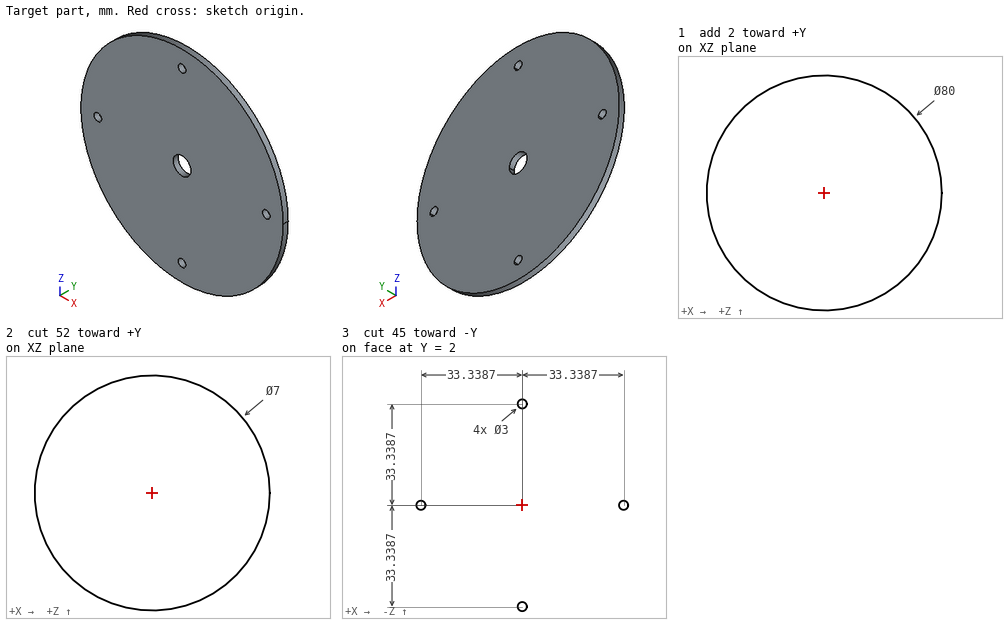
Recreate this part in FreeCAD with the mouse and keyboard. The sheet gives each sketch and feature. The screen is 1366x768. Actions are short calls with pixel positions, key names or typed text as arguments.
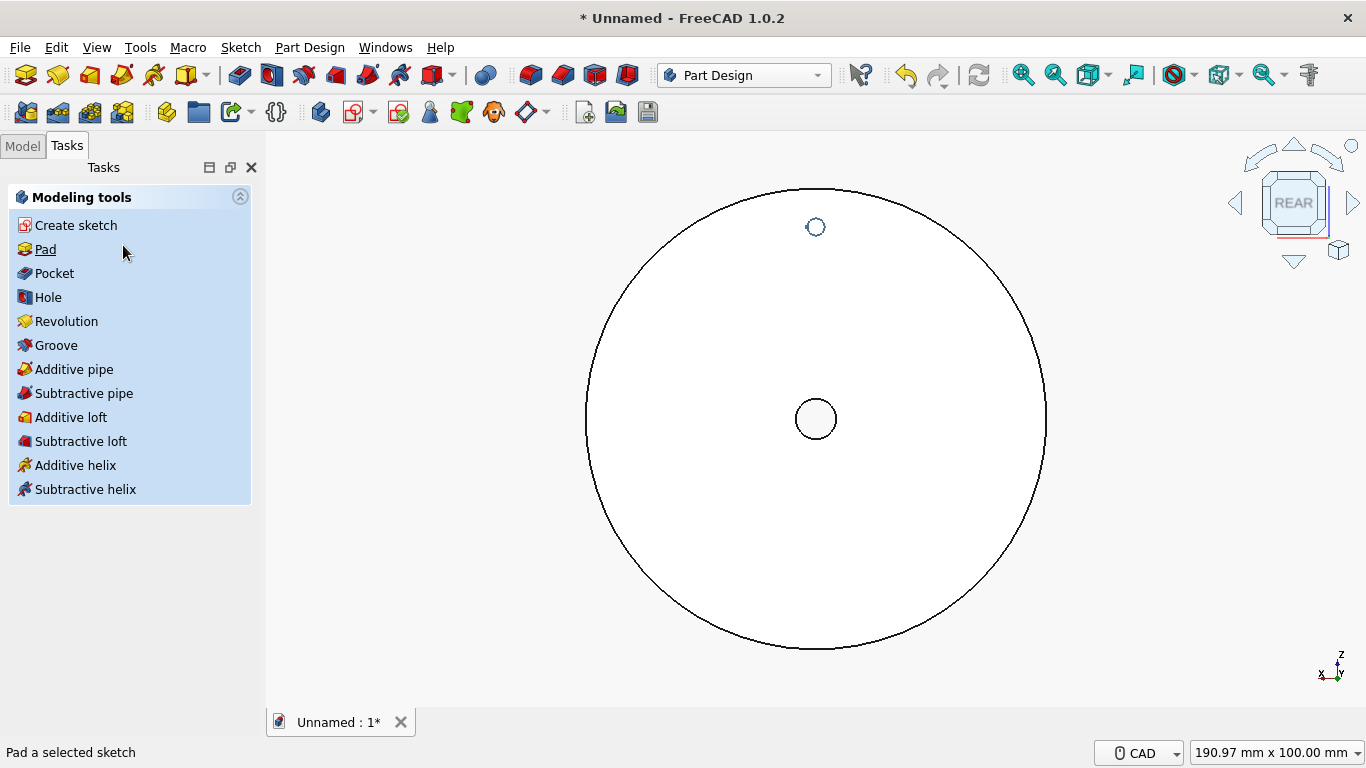
click(240, 76)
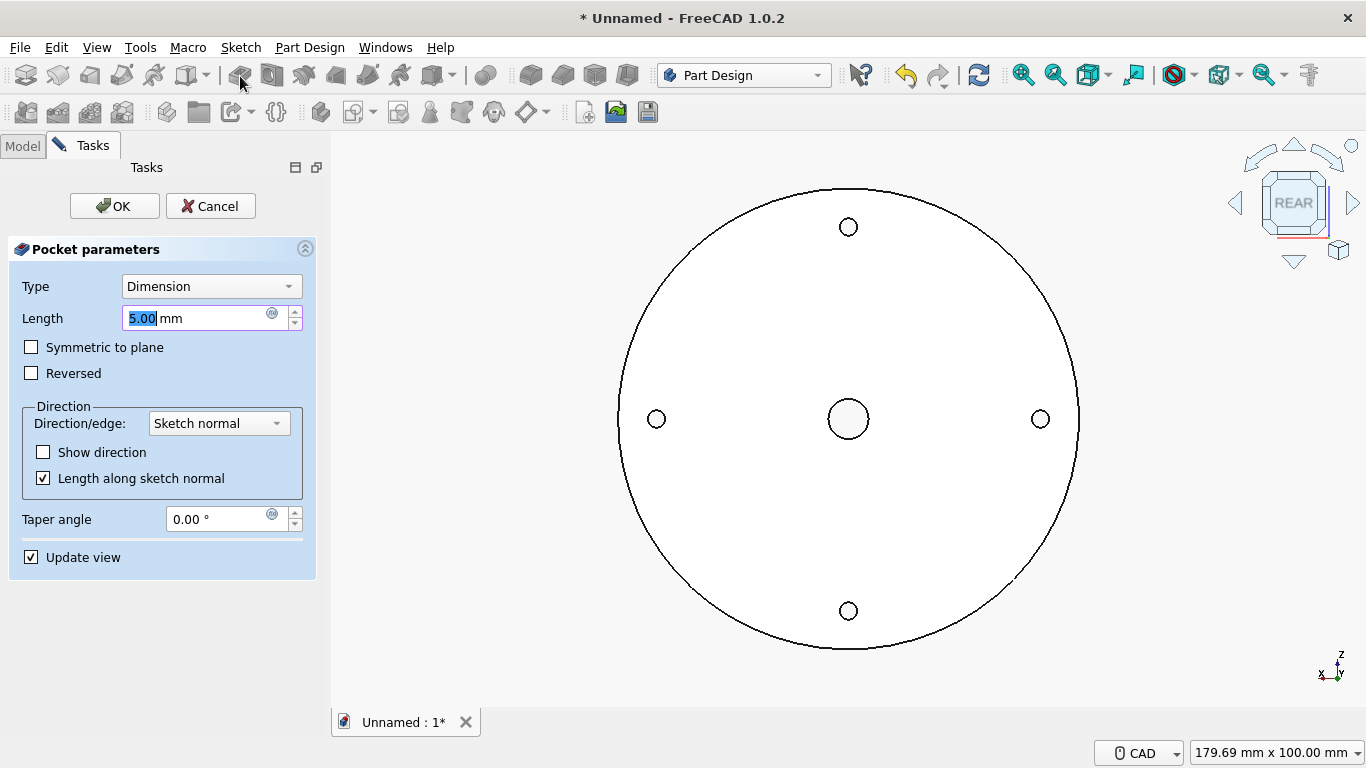
text(45)
key(Tab)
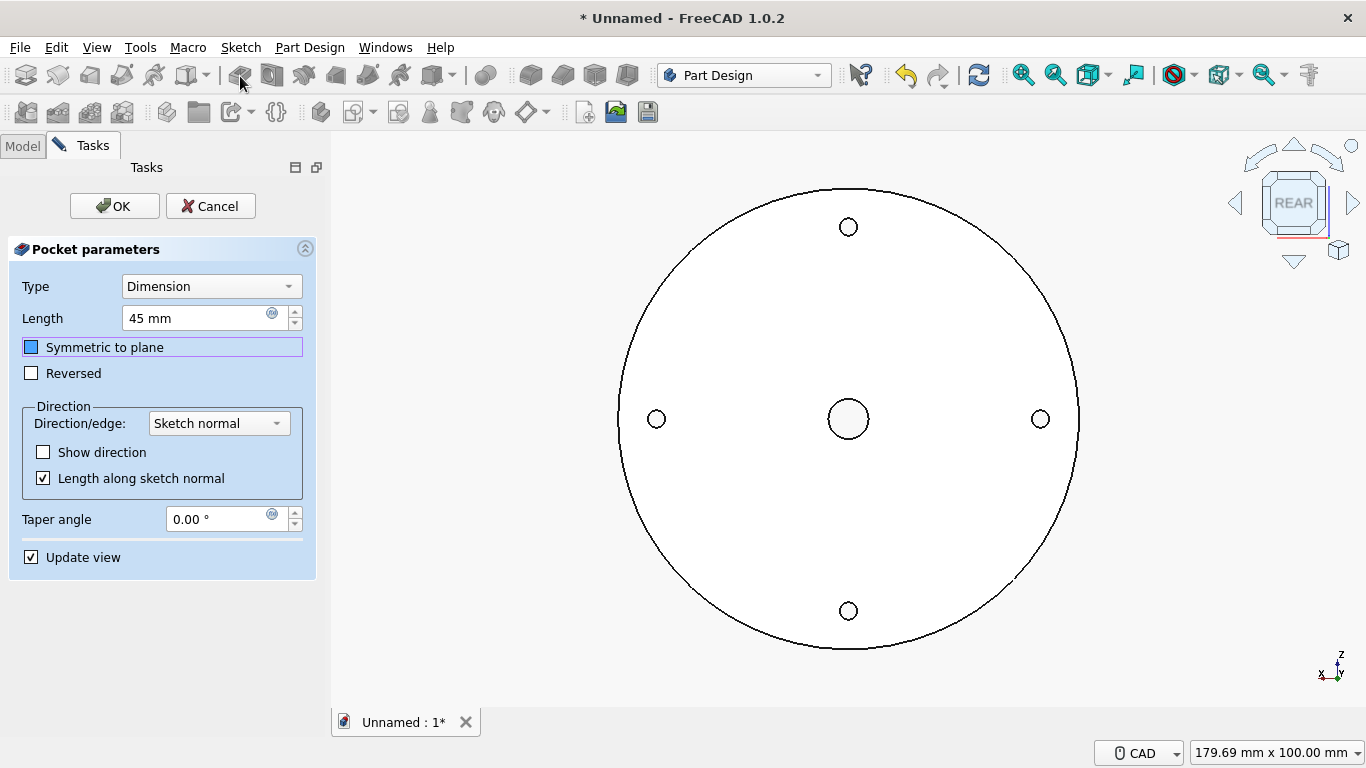
click(115, 206)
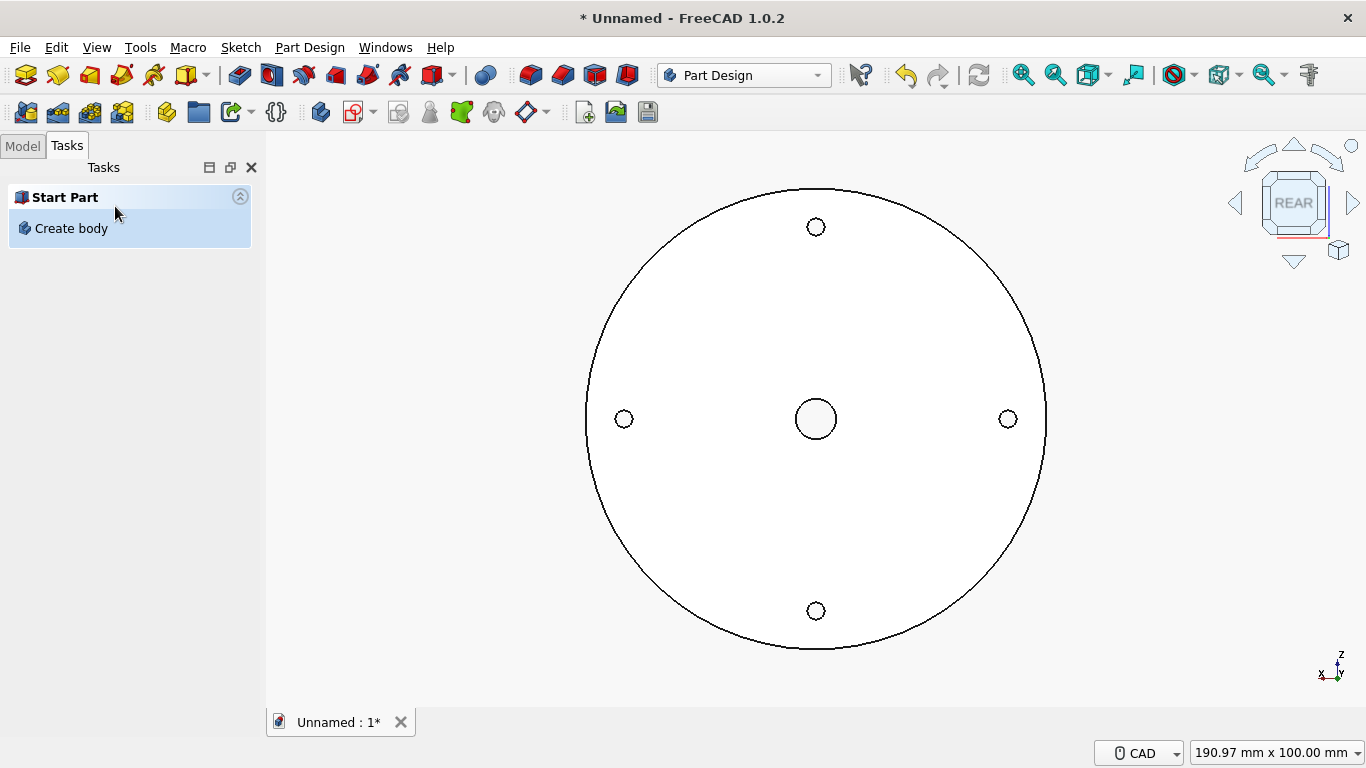
key(0)